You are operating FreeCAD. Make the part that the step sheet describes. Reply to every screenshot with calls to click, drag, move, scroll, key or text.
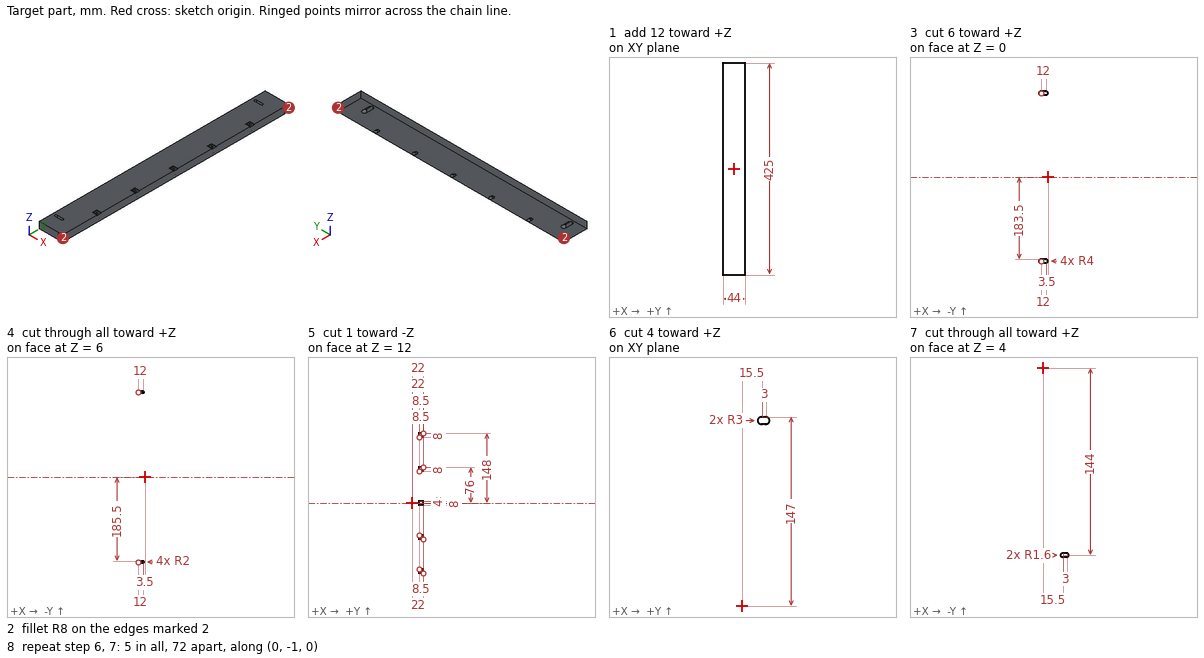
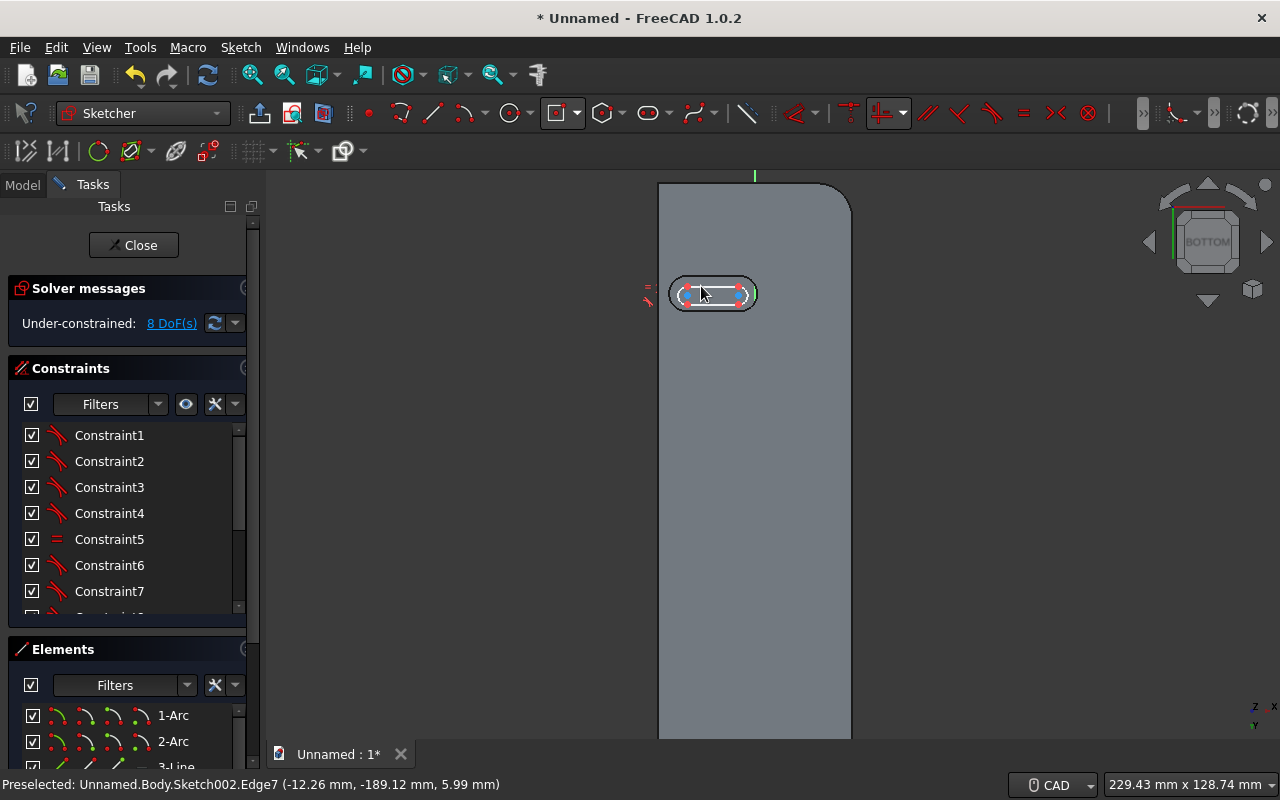
scroll(701, 286, down, 8)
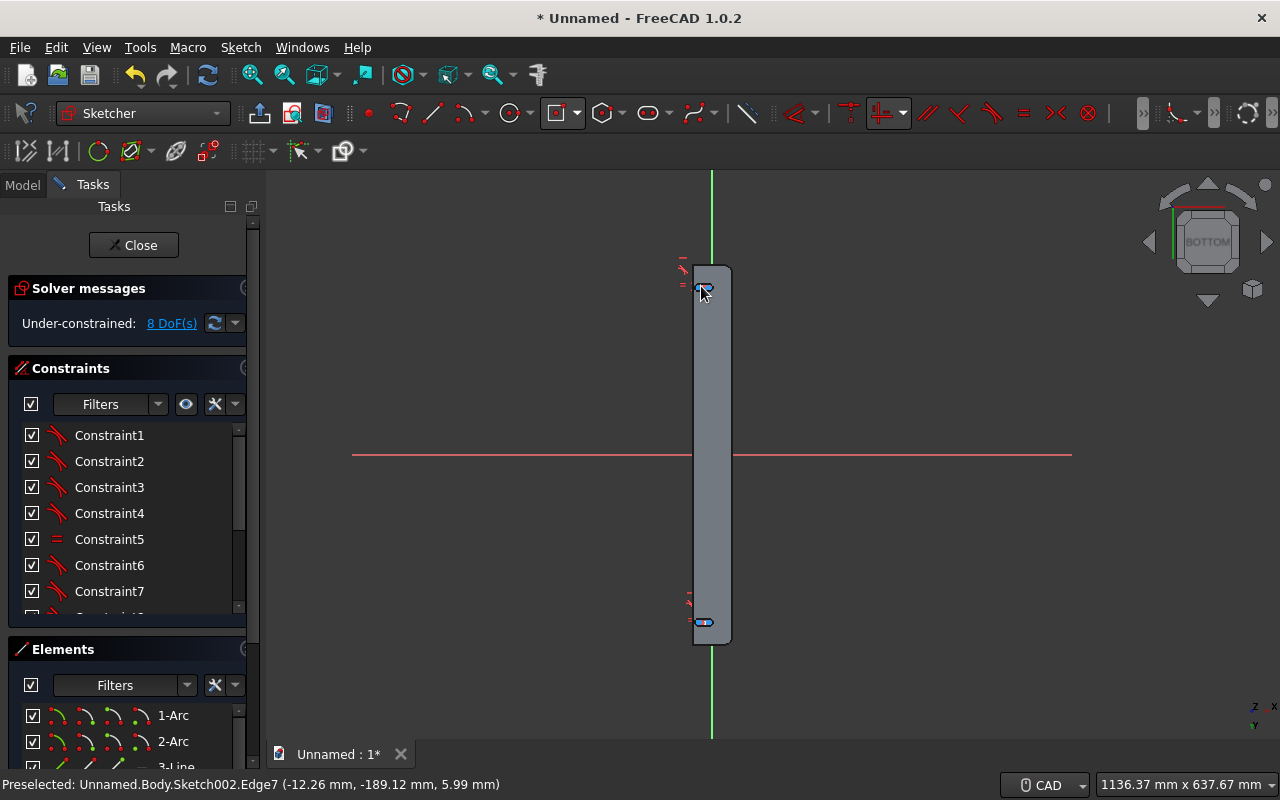
scroll(698, 623, up, 13)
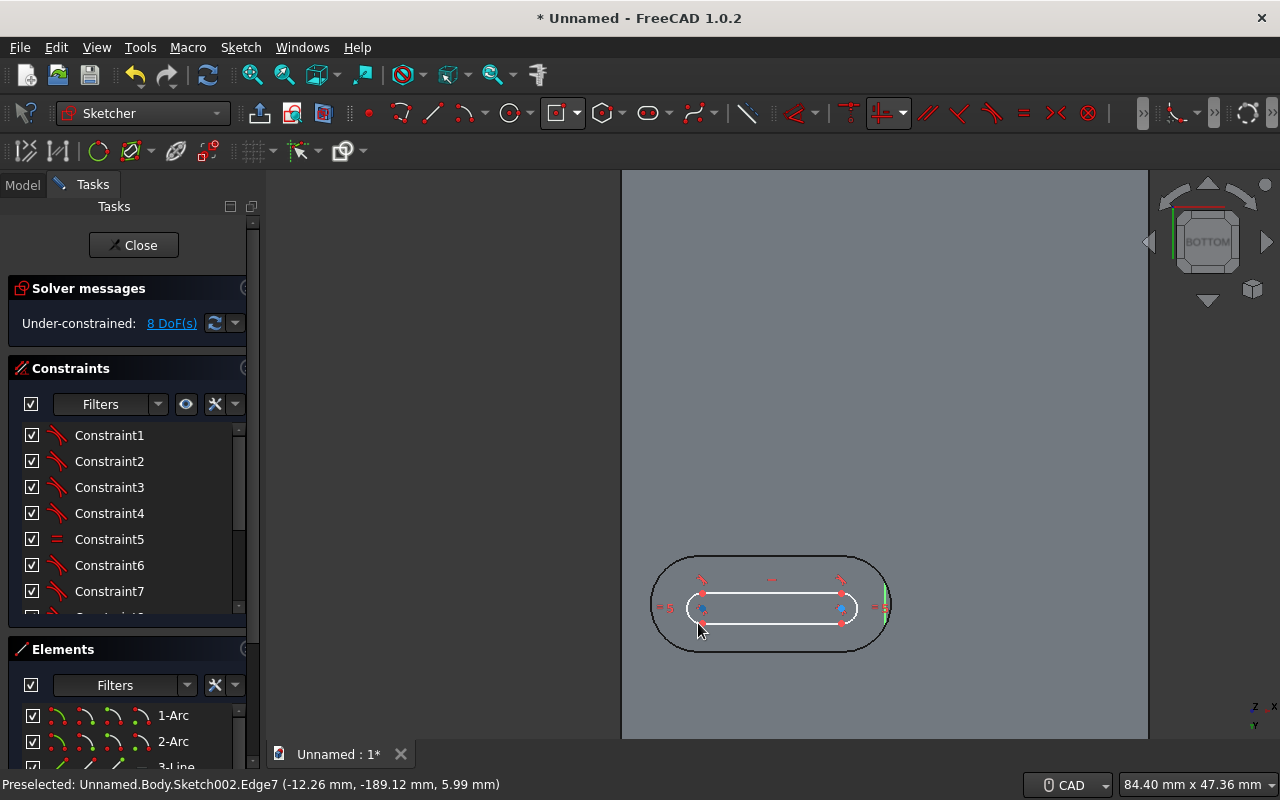
click(687, 609)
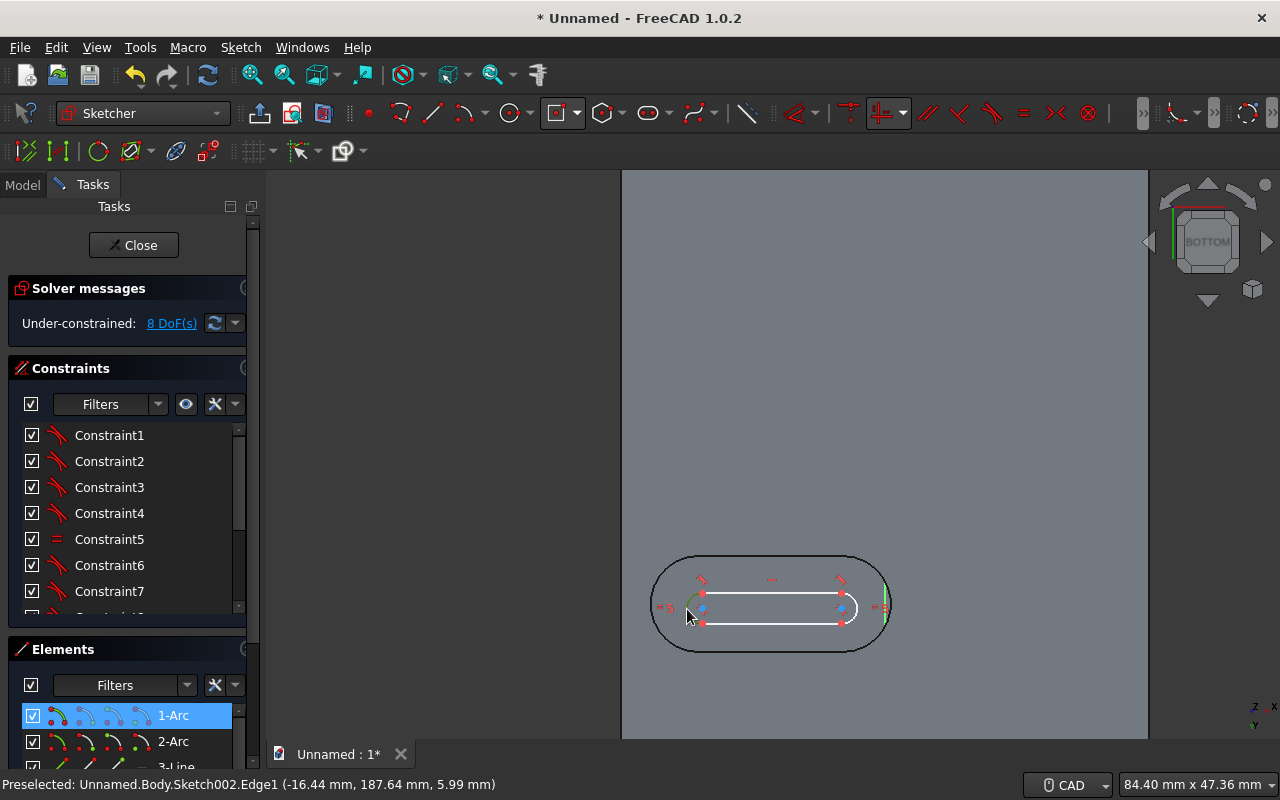
scroll(698, 623, down, 13)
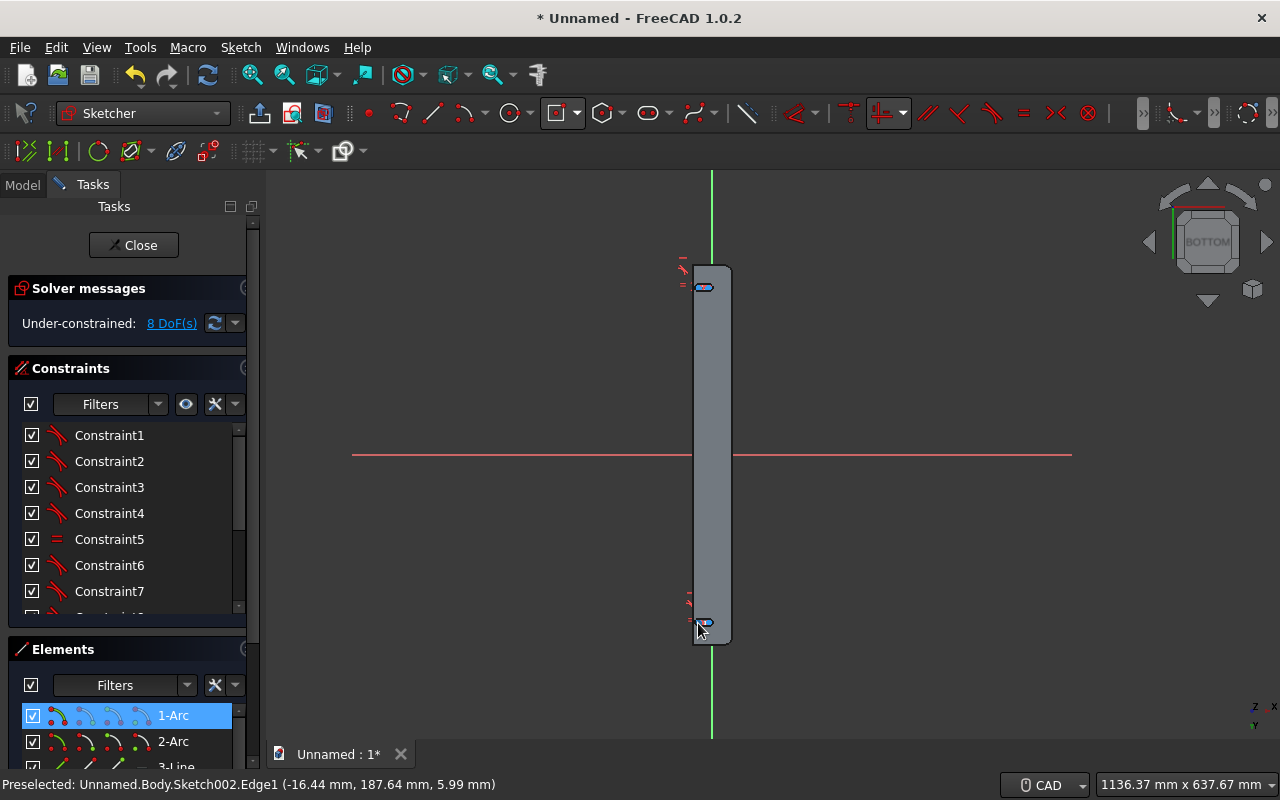
scroll(697, 287, up, 11)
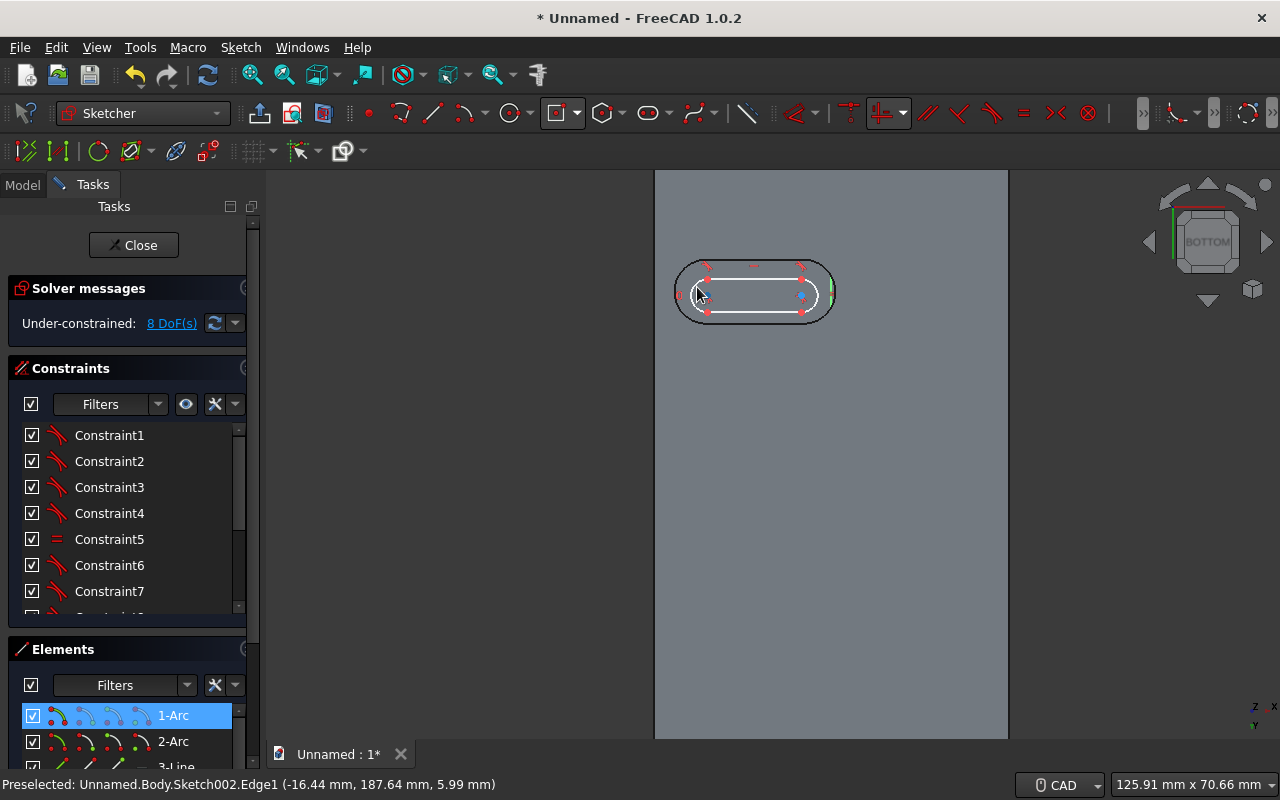
click(694, 286)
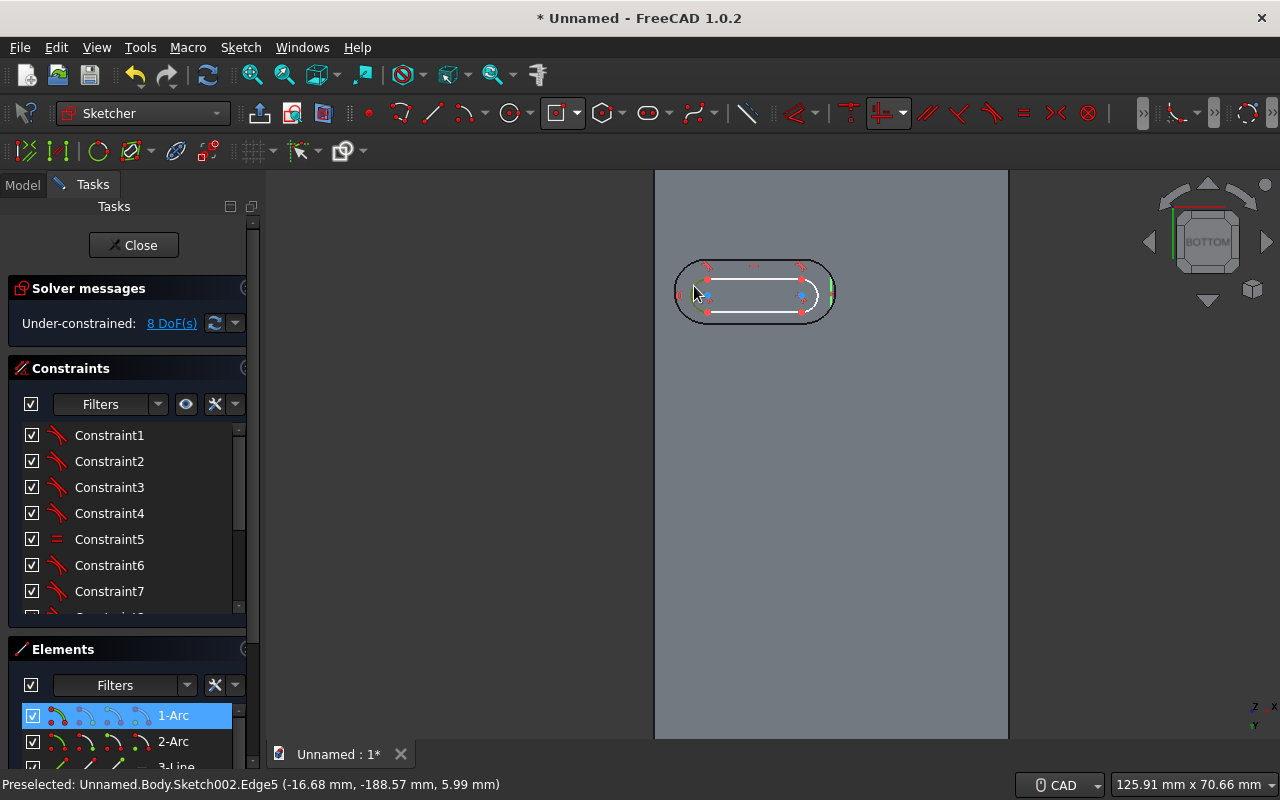
click(1024, 114)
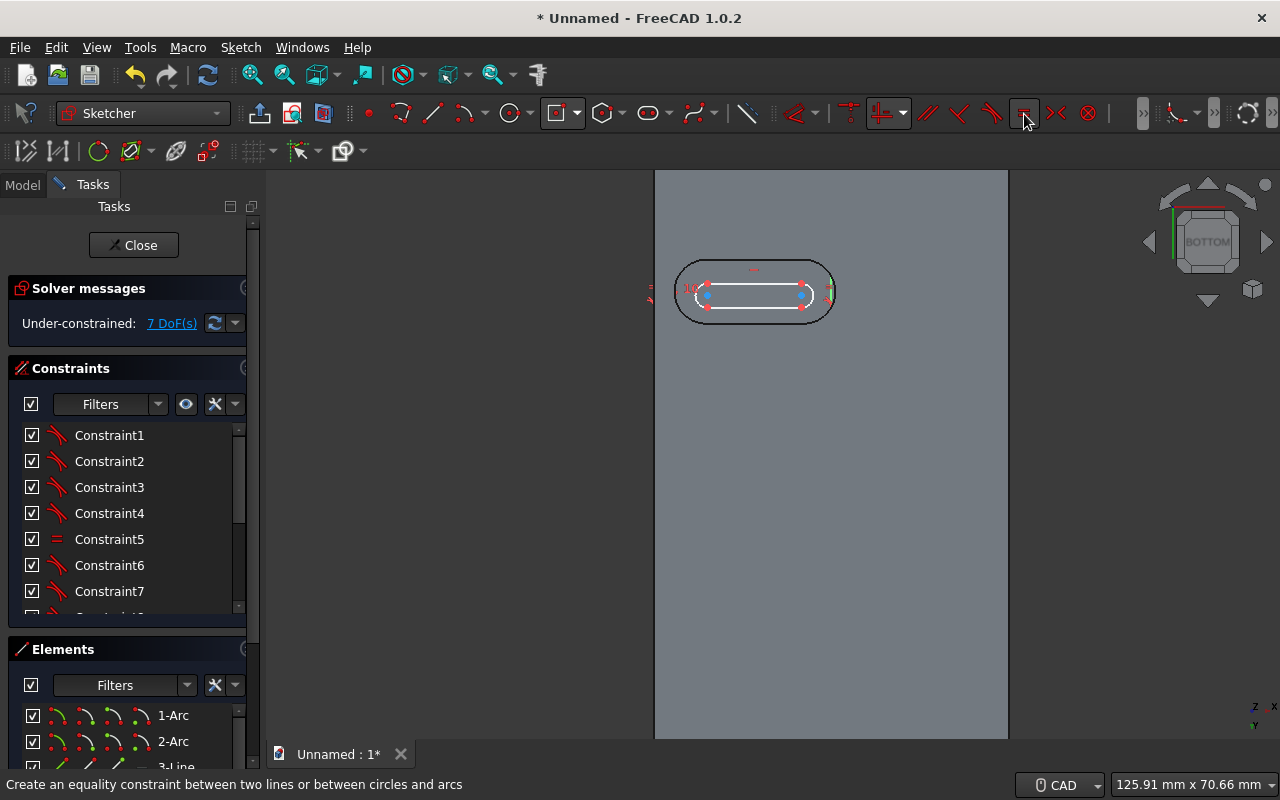
scroll(697, 287, down, 11)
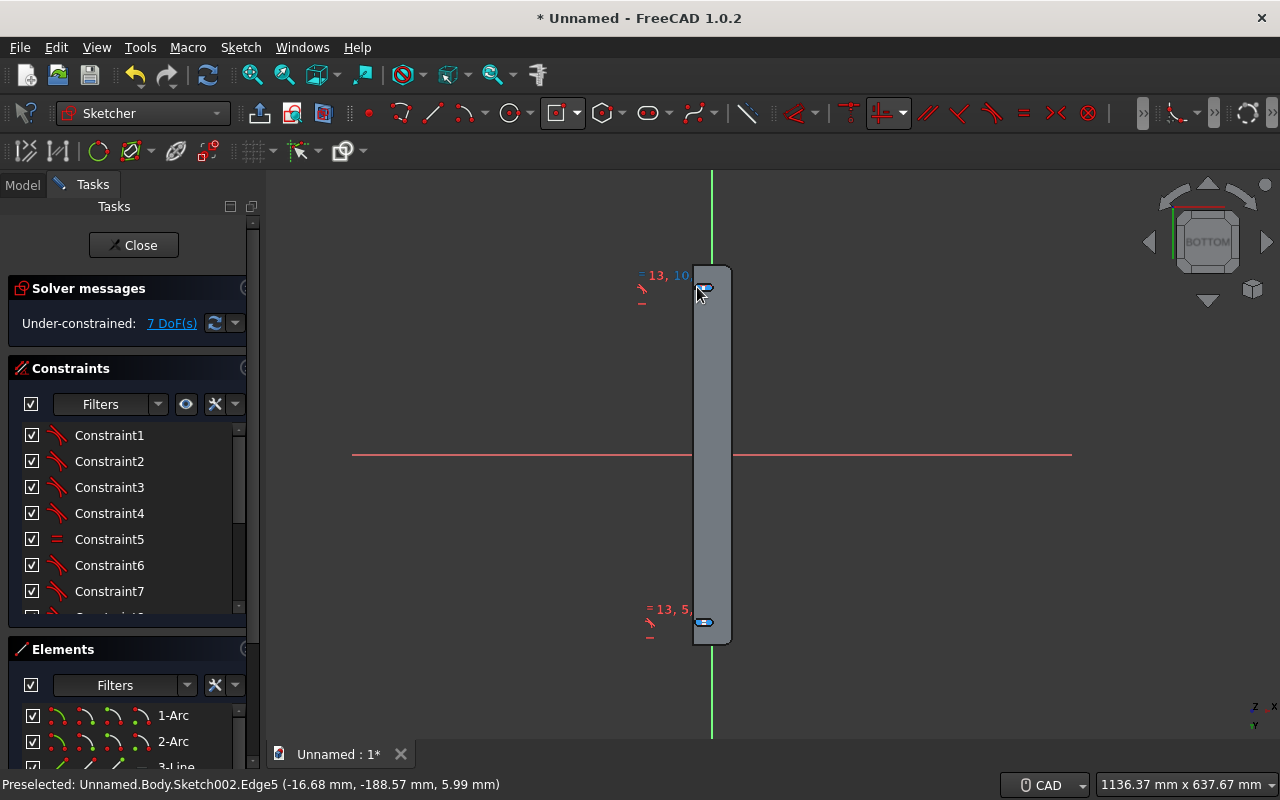
scroll(699, 623, up, 12)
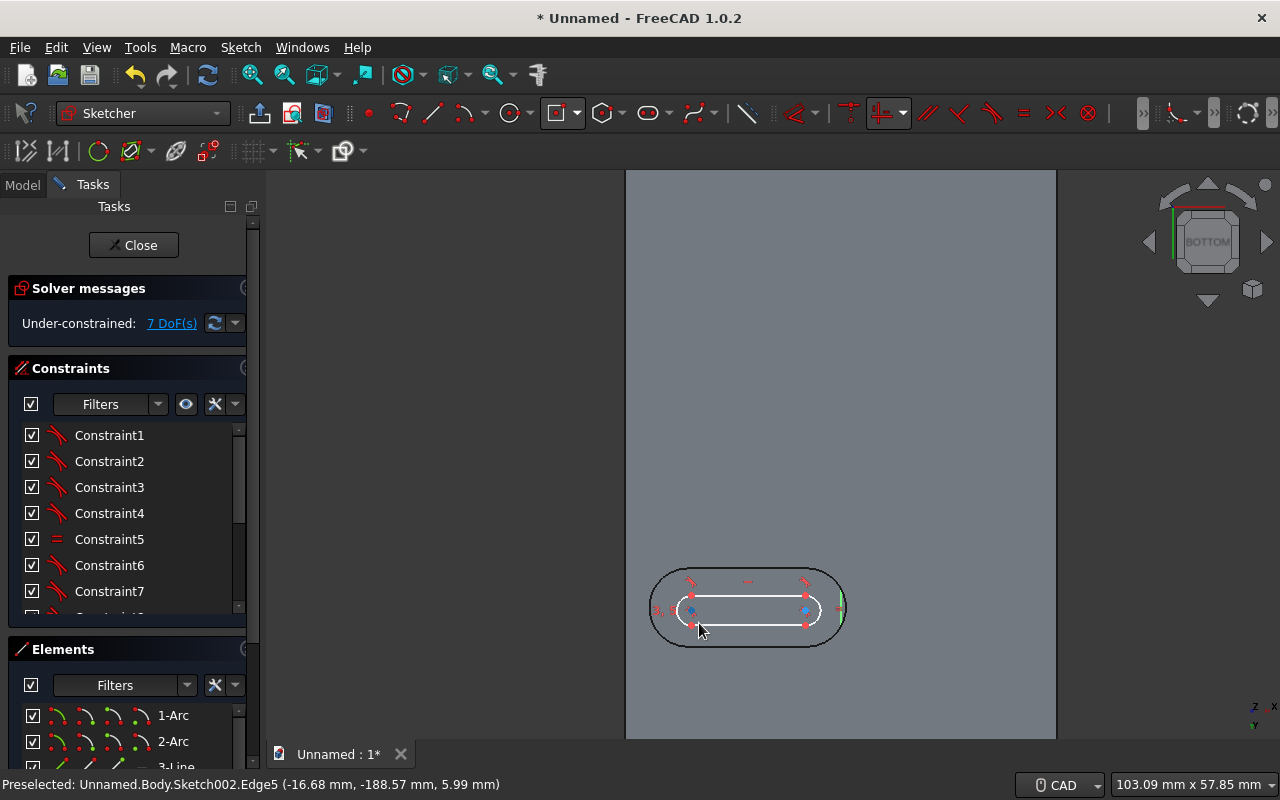
click(692, 611)